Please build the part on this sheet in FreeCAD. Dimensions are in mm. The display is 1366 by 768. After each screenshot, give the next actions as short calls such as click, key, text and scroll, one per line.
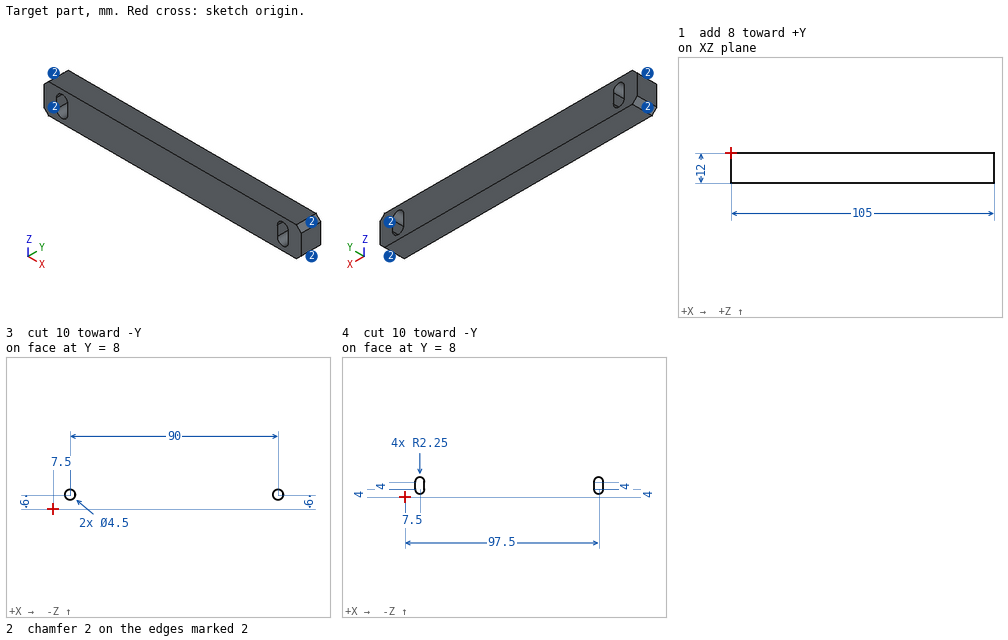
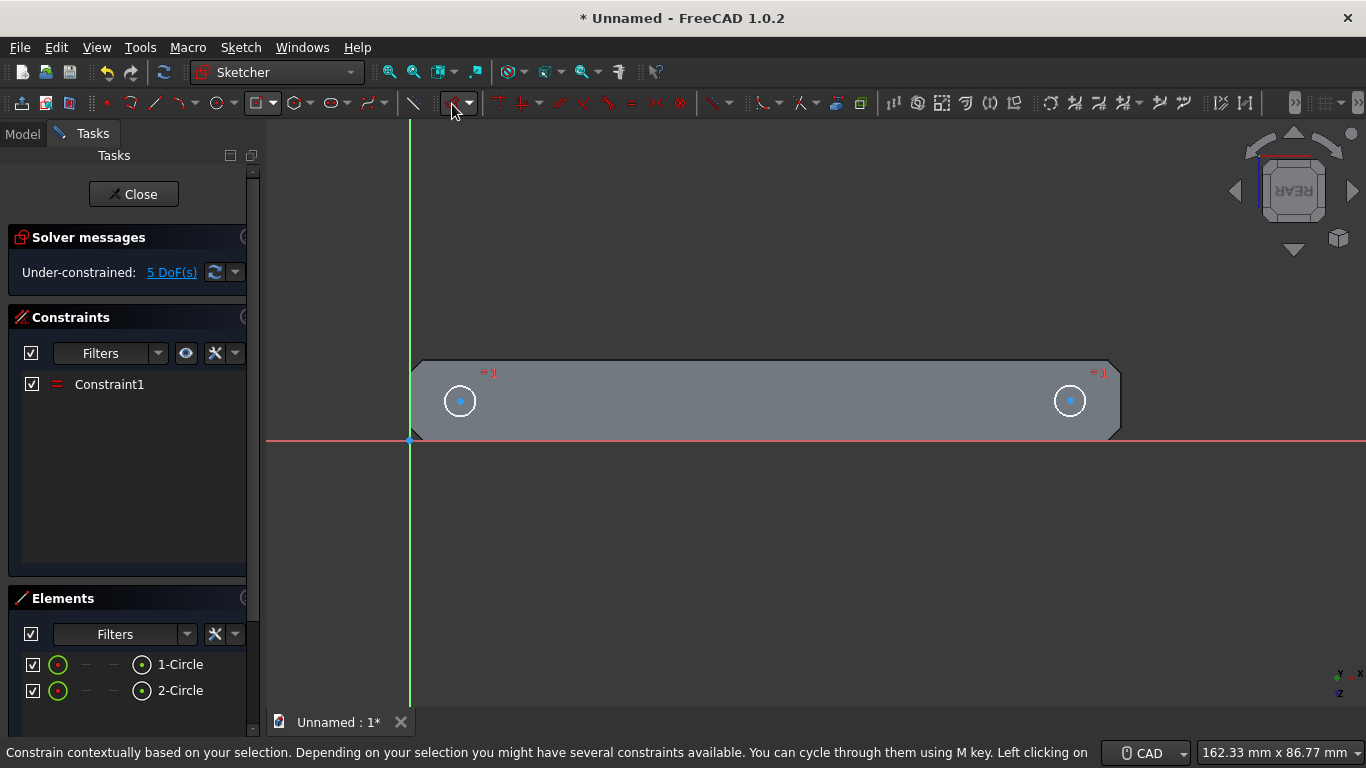
scroll(471, 391, up, 2)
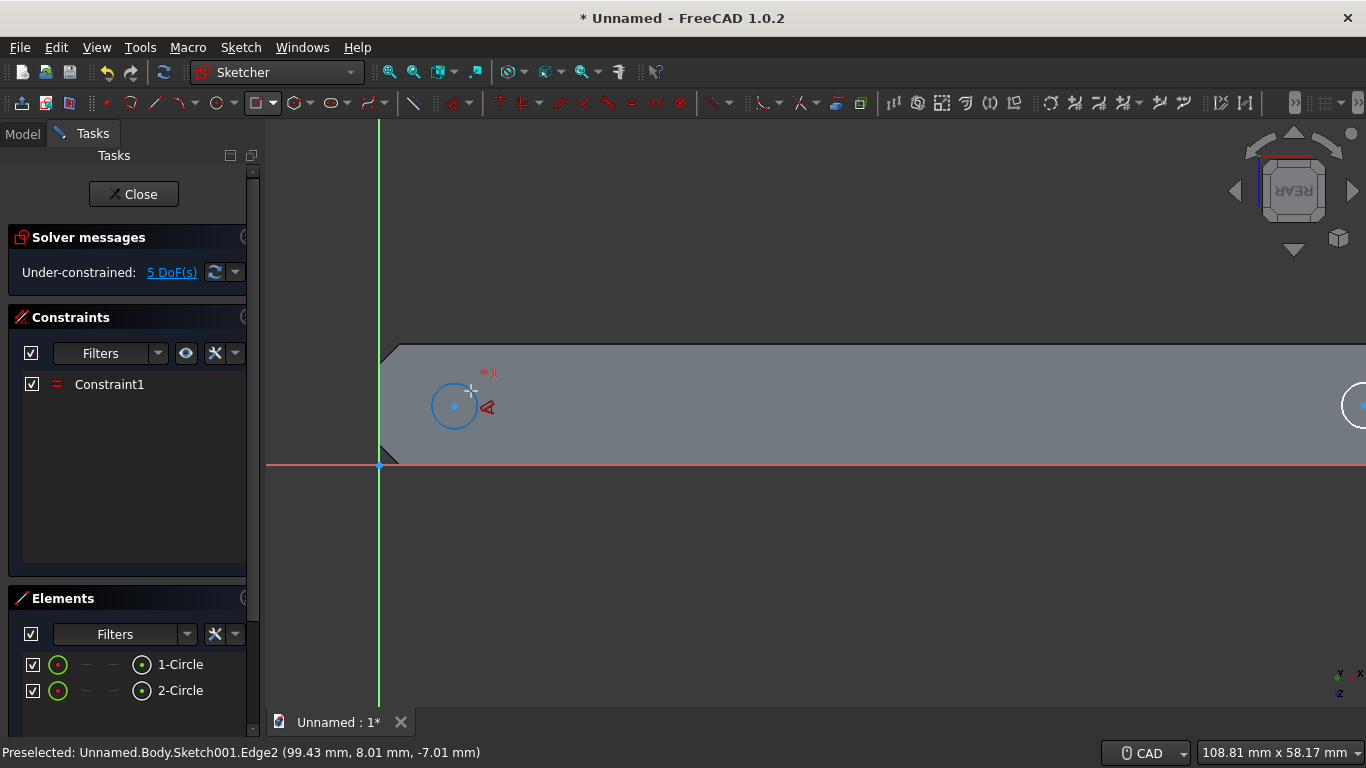
click(471, 390)
click(494, 367)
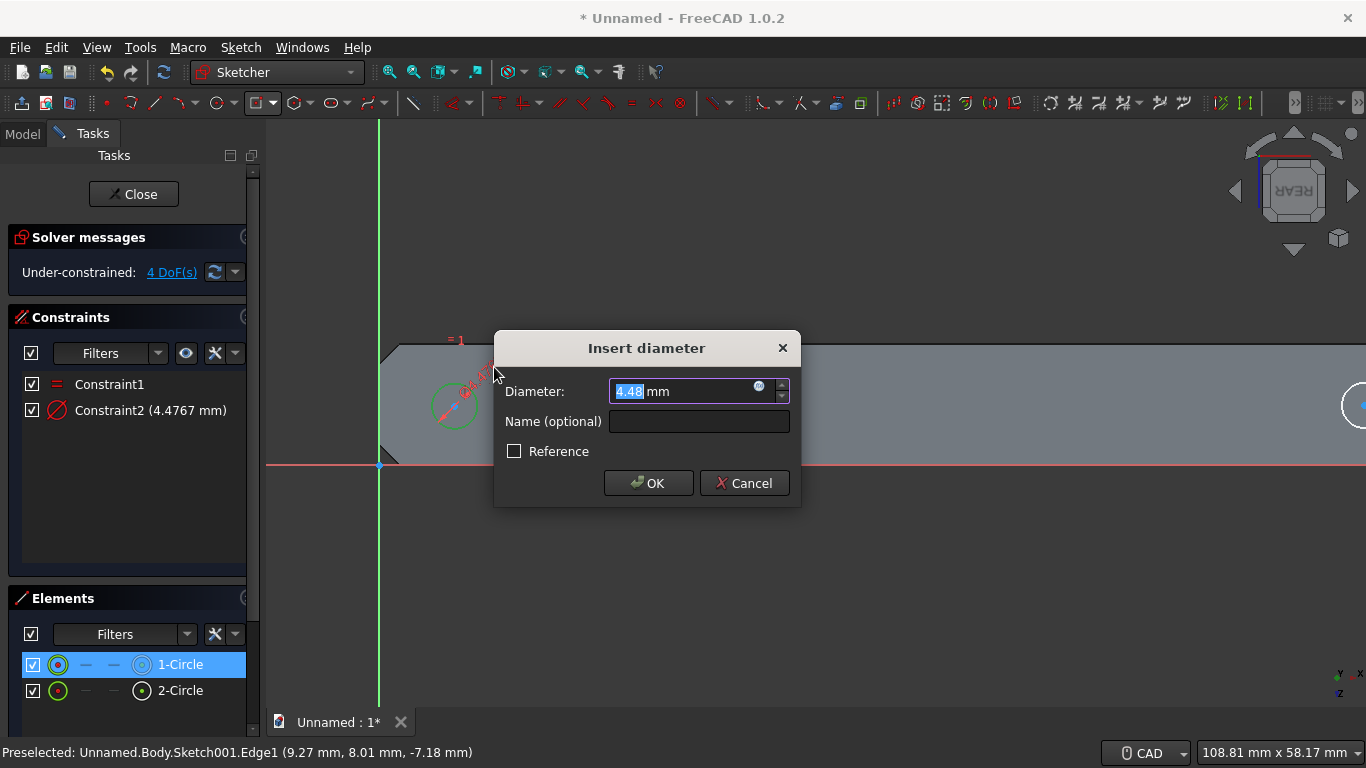
text(4.5)
key(Return)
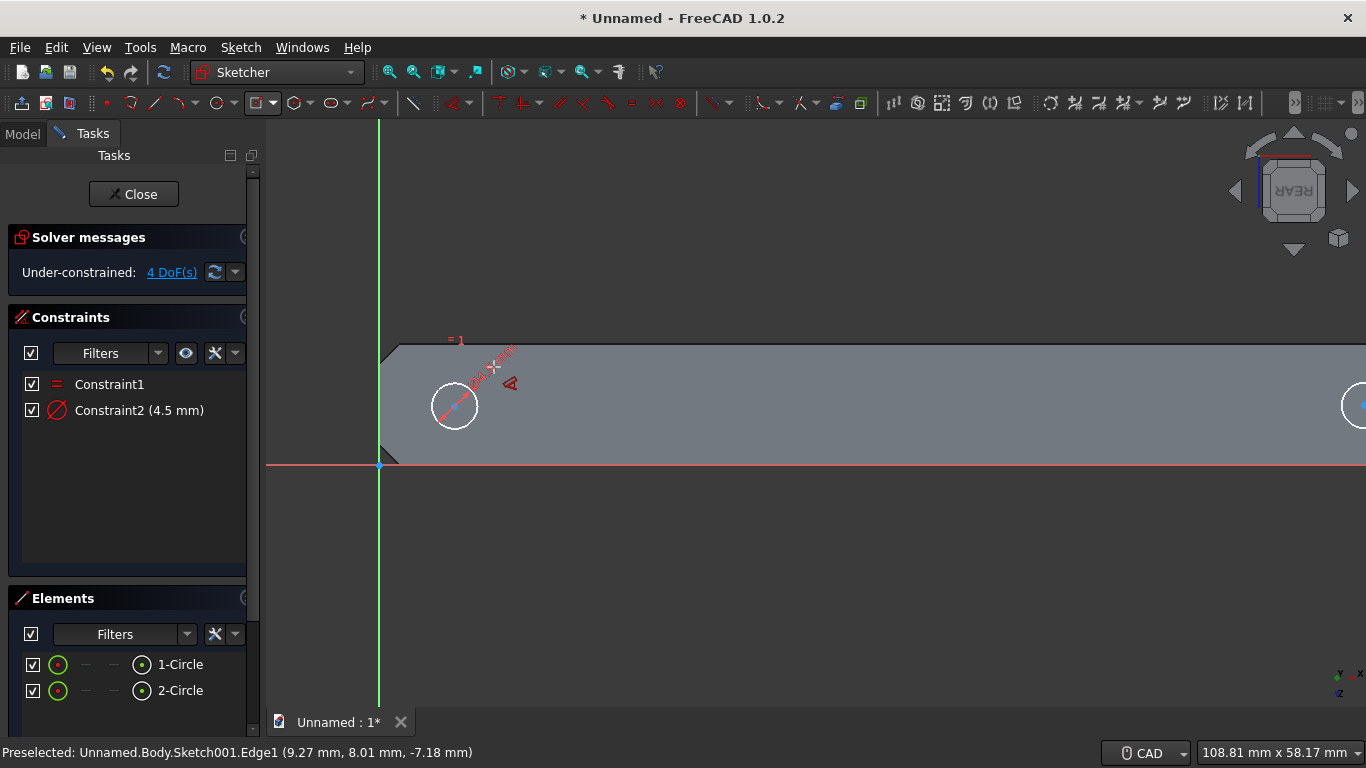
click(455, 406)
click(345, 436)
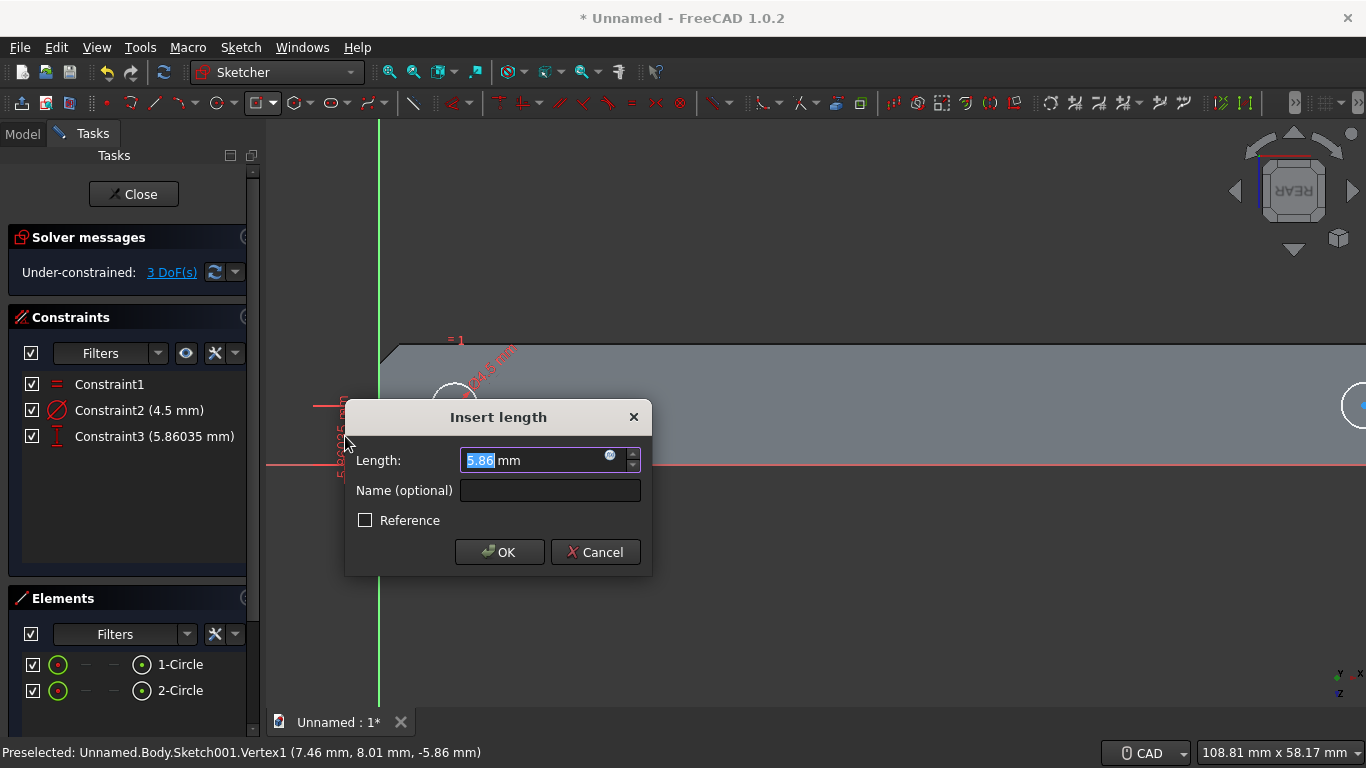
text(6)
key(Return)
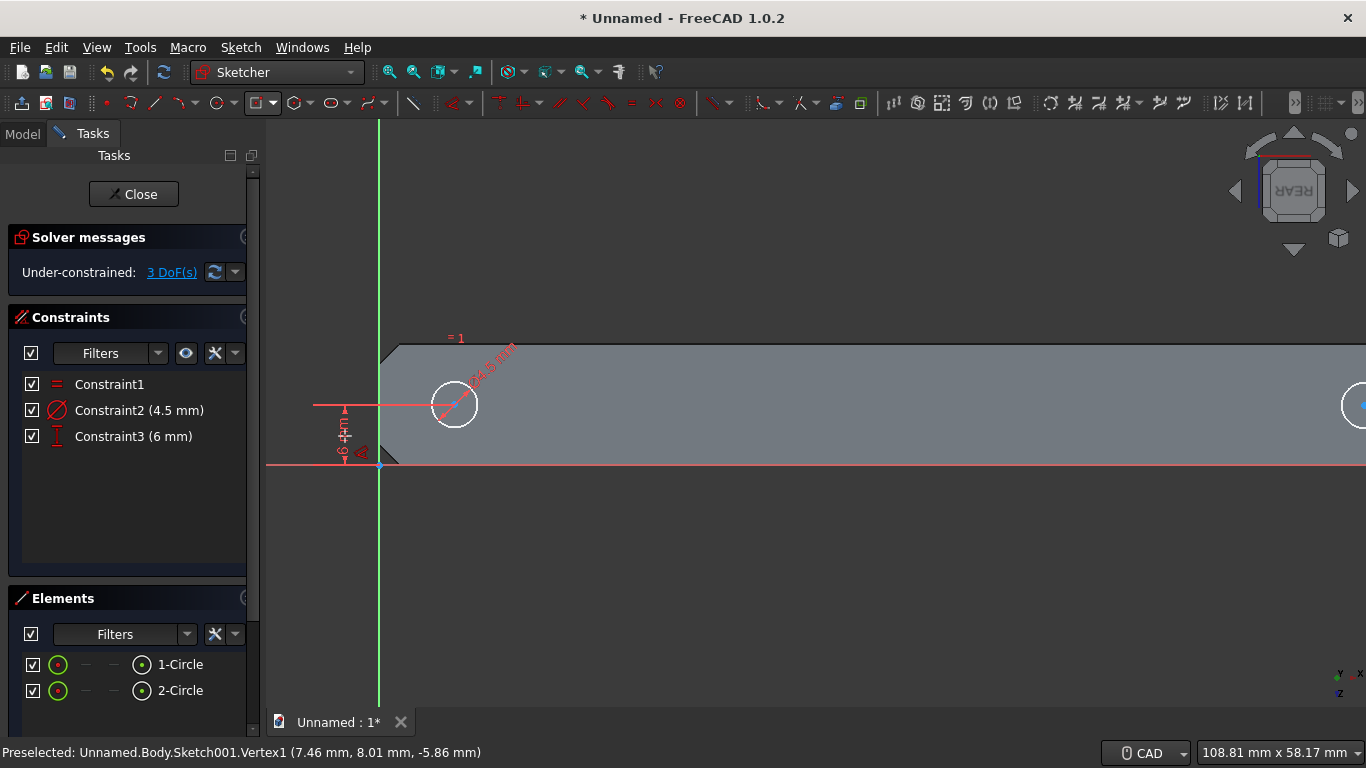
scroll(471, 391, down, 2)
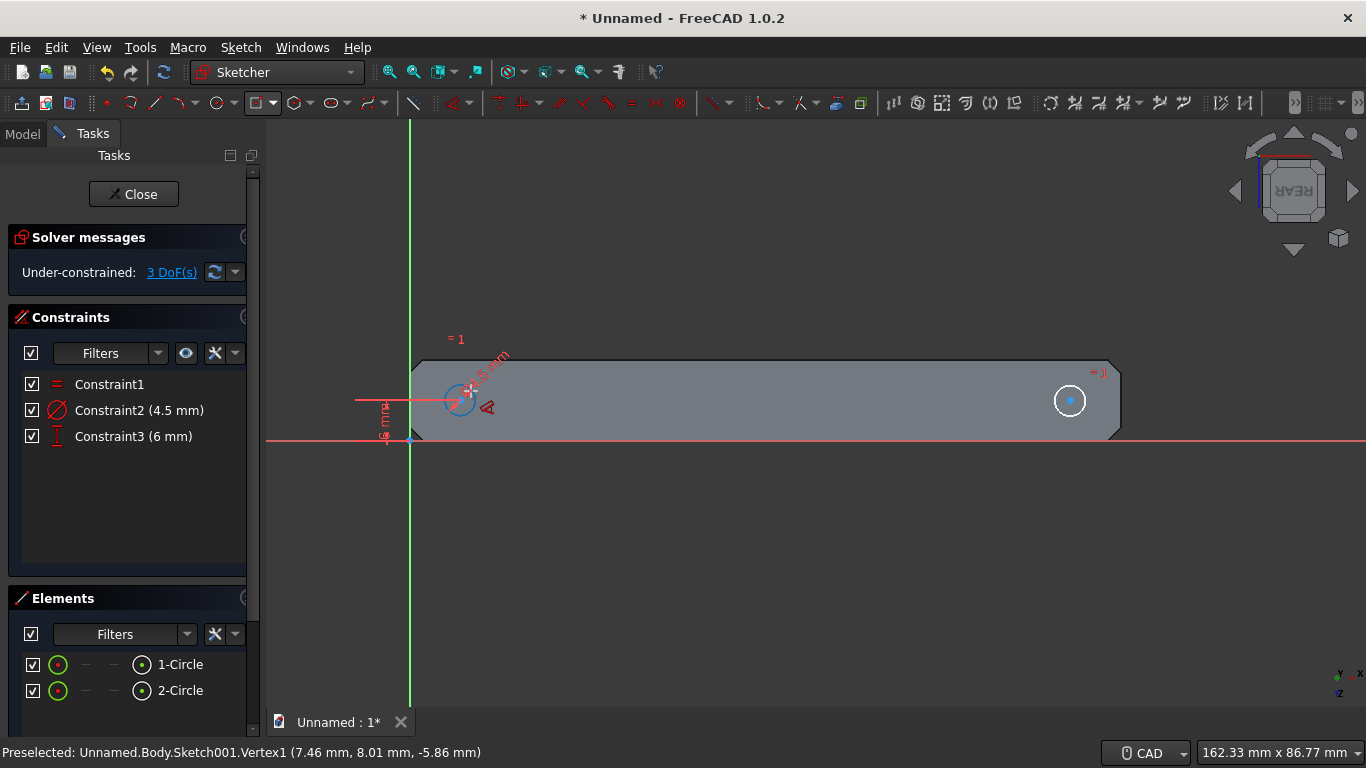
click(1070, 401)
click(1104, 421)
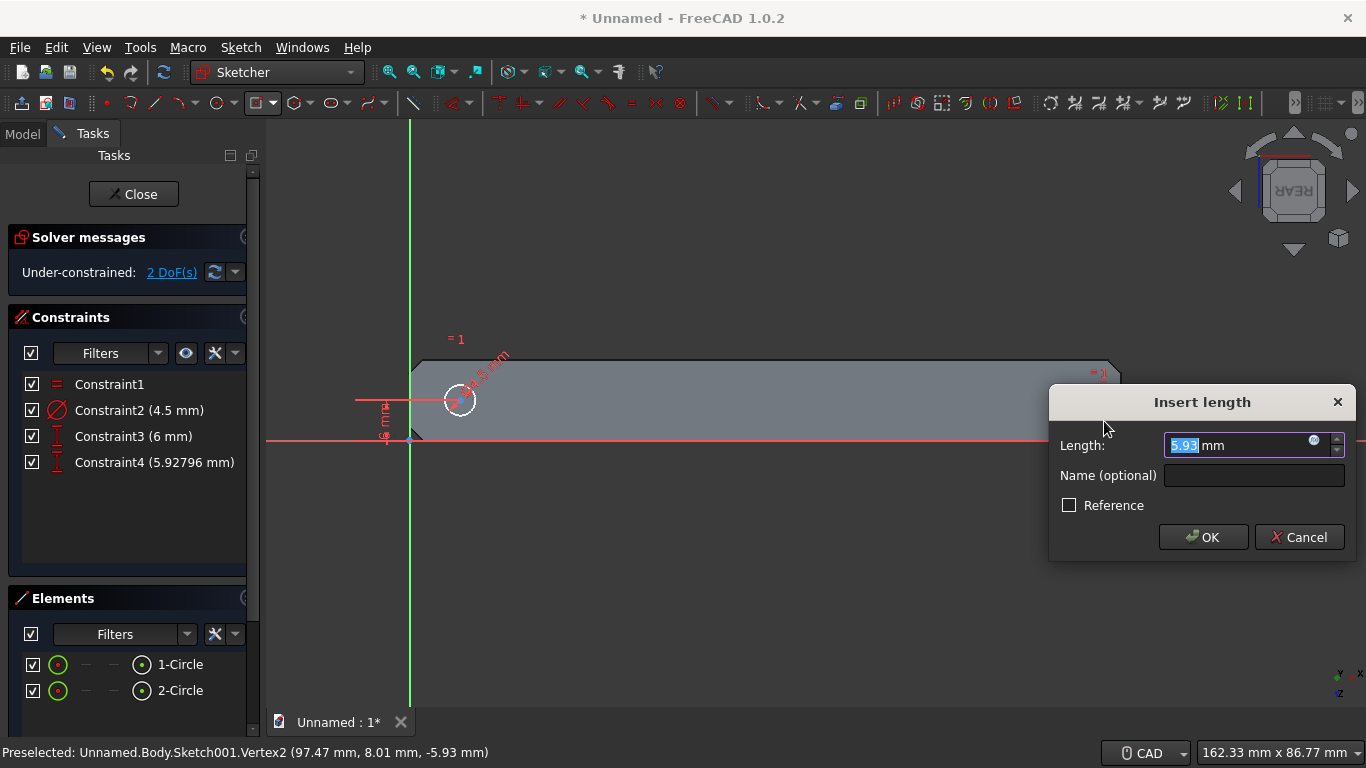
text(6)
key(Return)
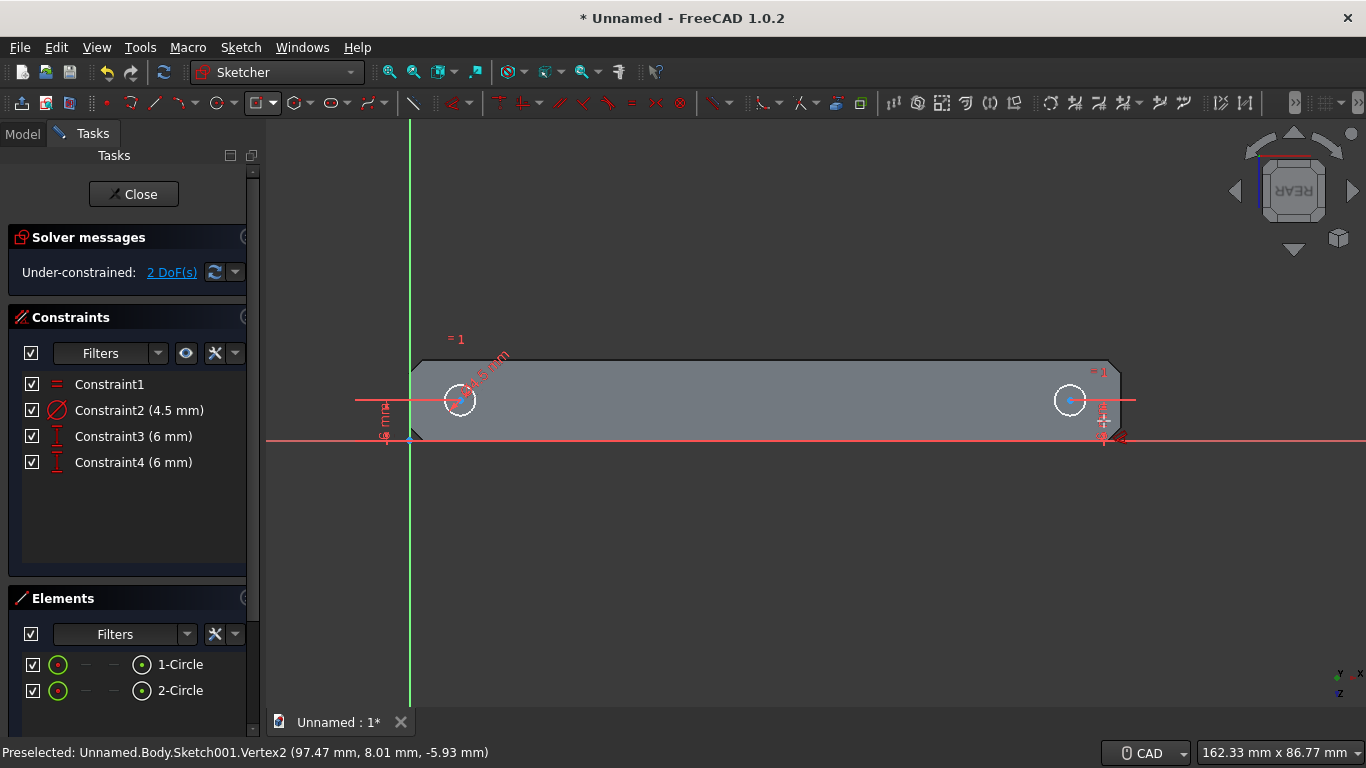
click(460, 400)
click(435, 475)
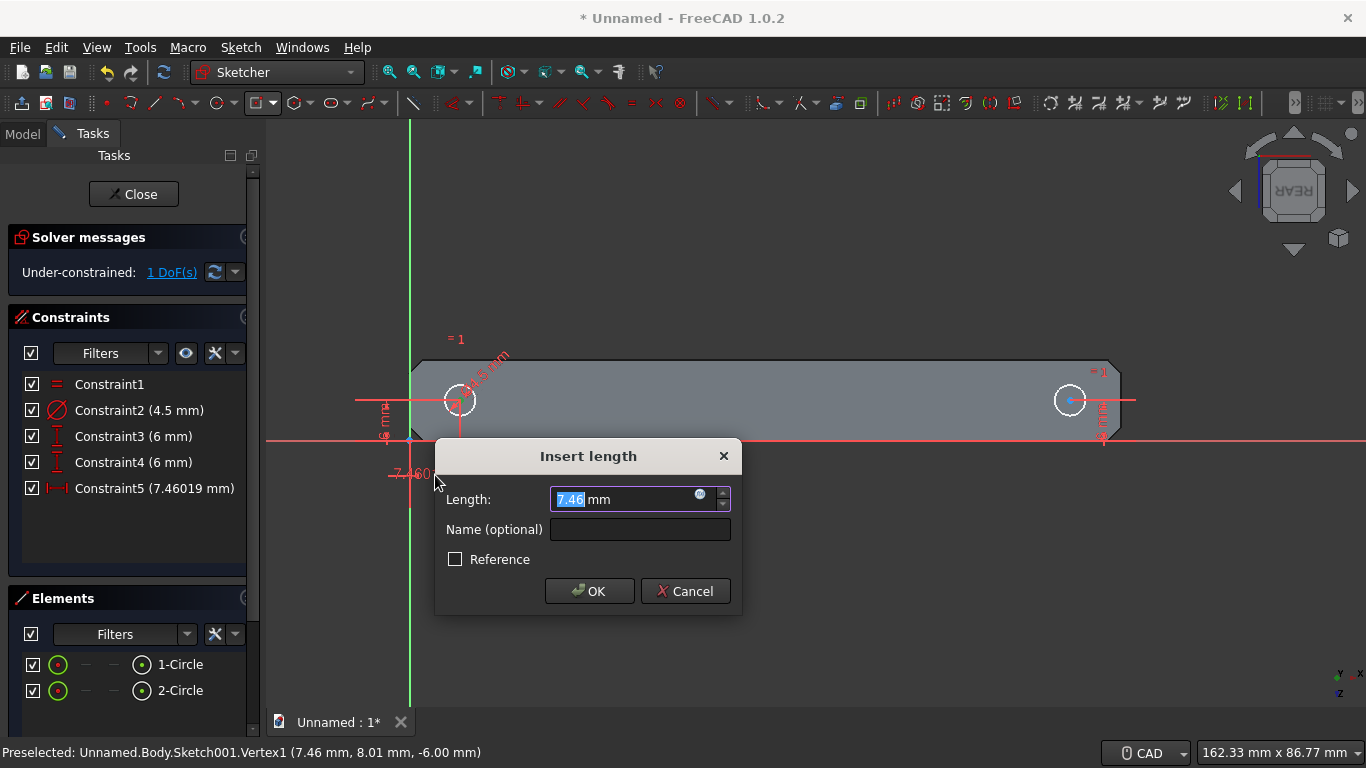
text(7.5)
key(Return)